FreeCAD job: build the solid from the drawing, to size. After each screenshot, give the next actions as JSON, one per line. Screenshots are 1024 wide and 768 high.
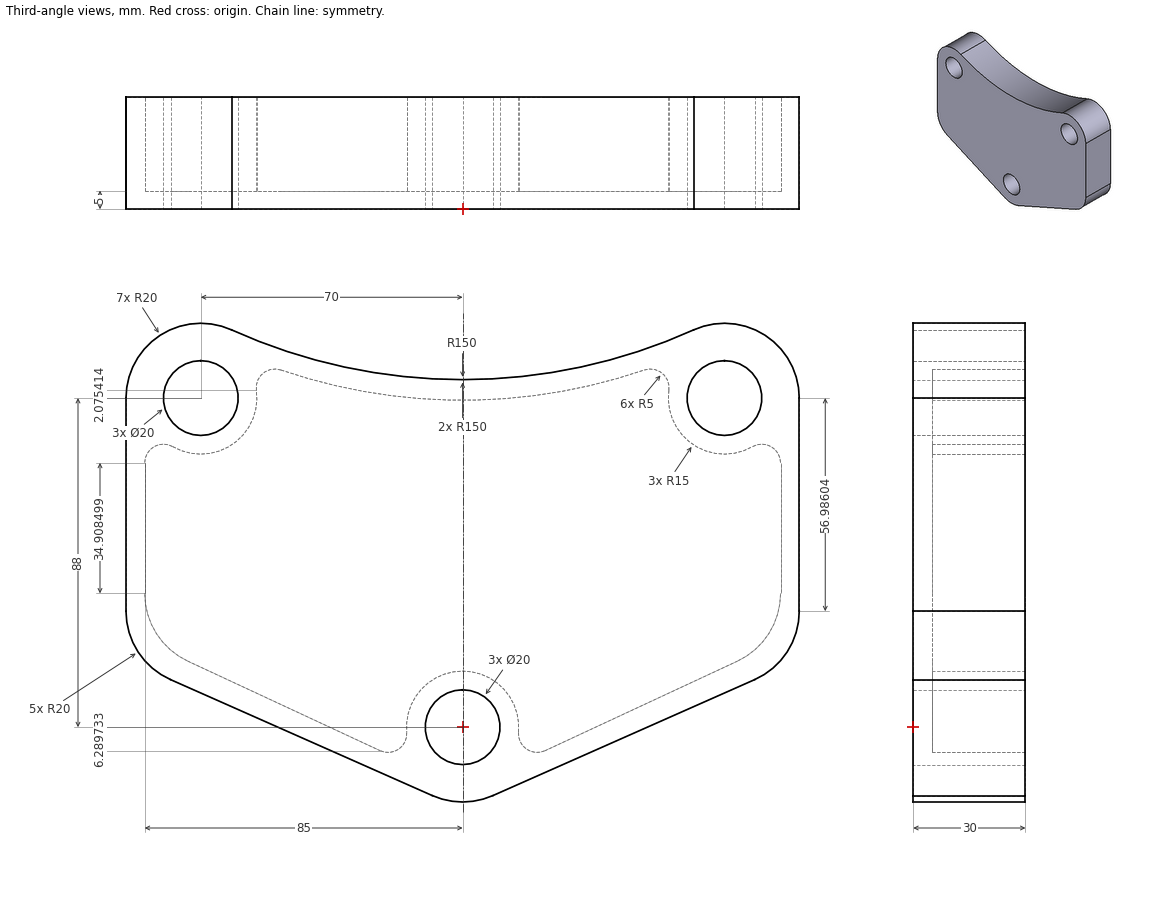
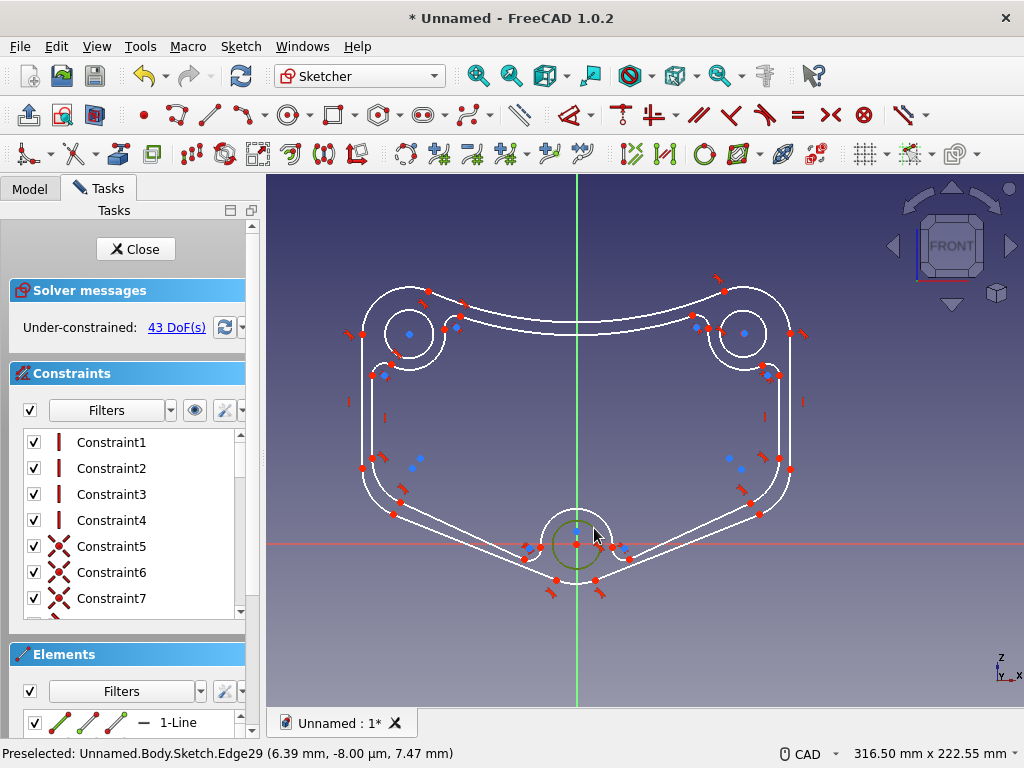
{"action": "left_click", "coordinate": [576, 584]}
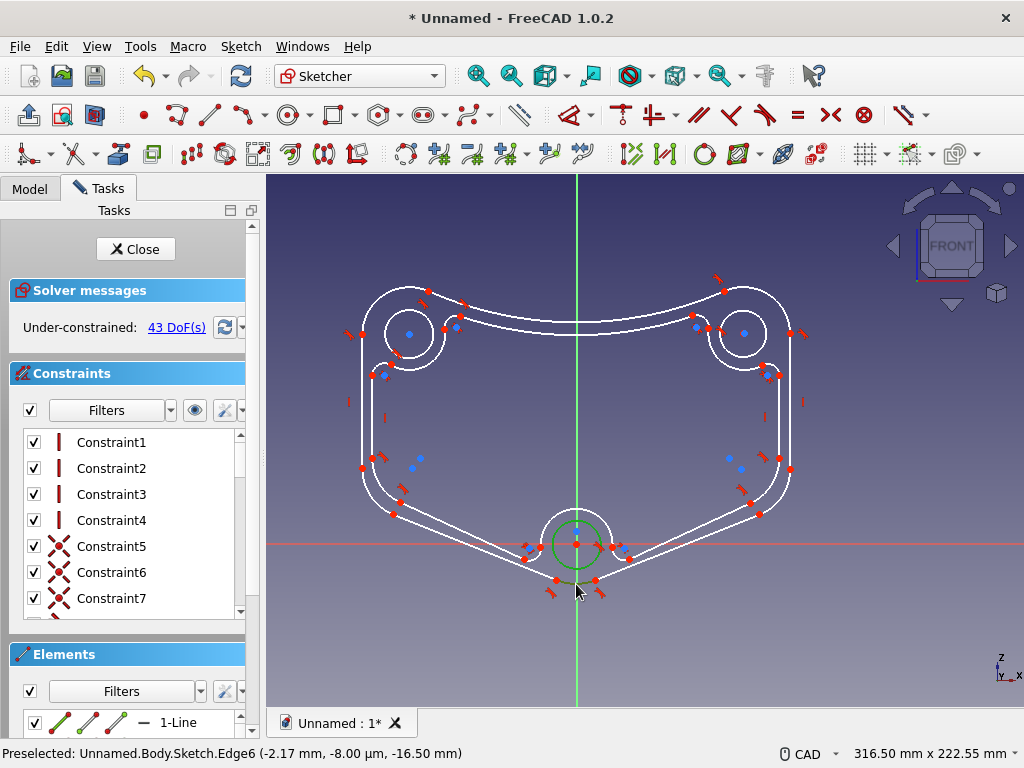
{"action": "left_click", "coordinate": [621, 116]}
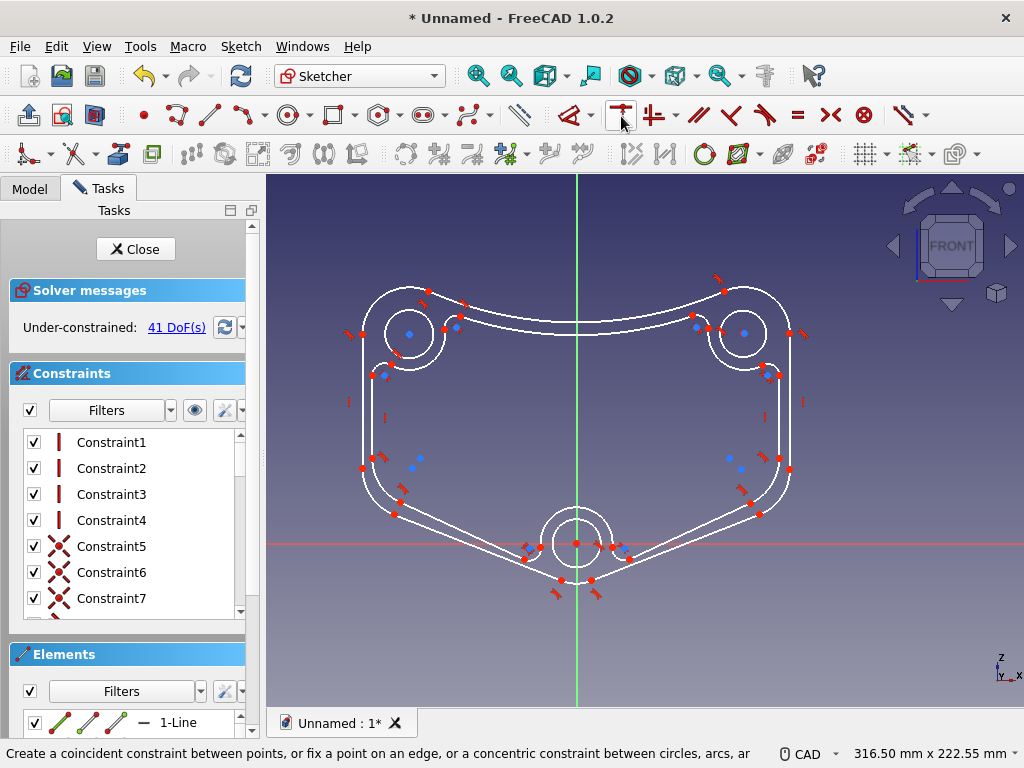
{"action": "left_click", "coordinate": [426, 317]}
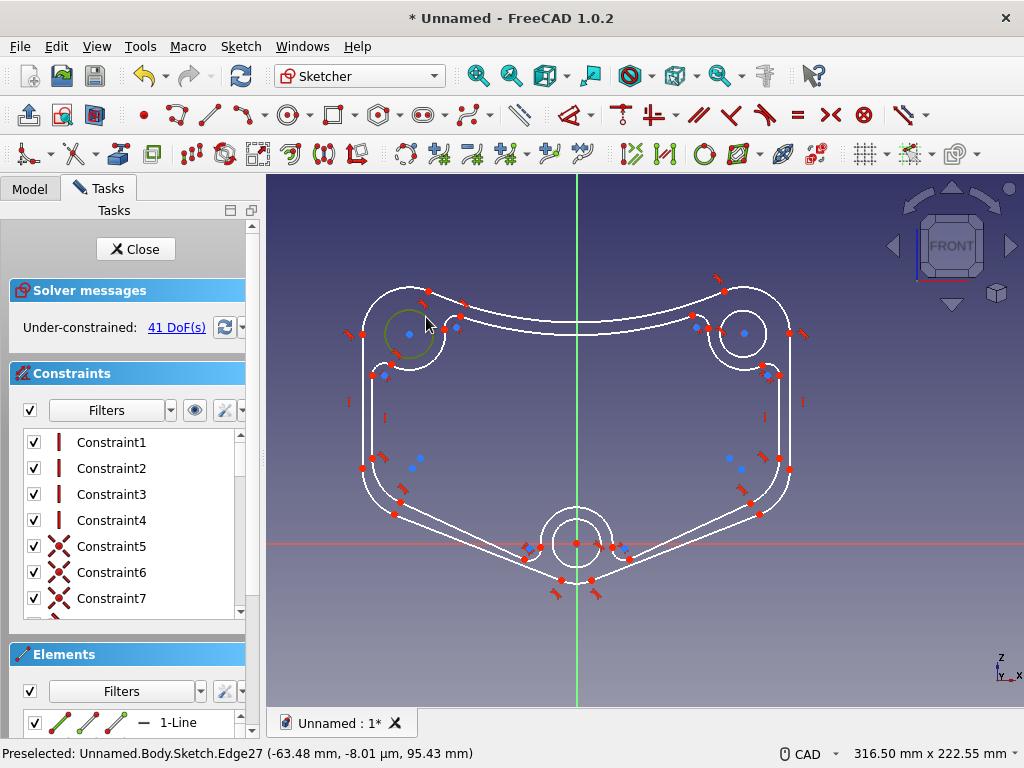
{"action": "left_click", "coordinate": [401, 288]}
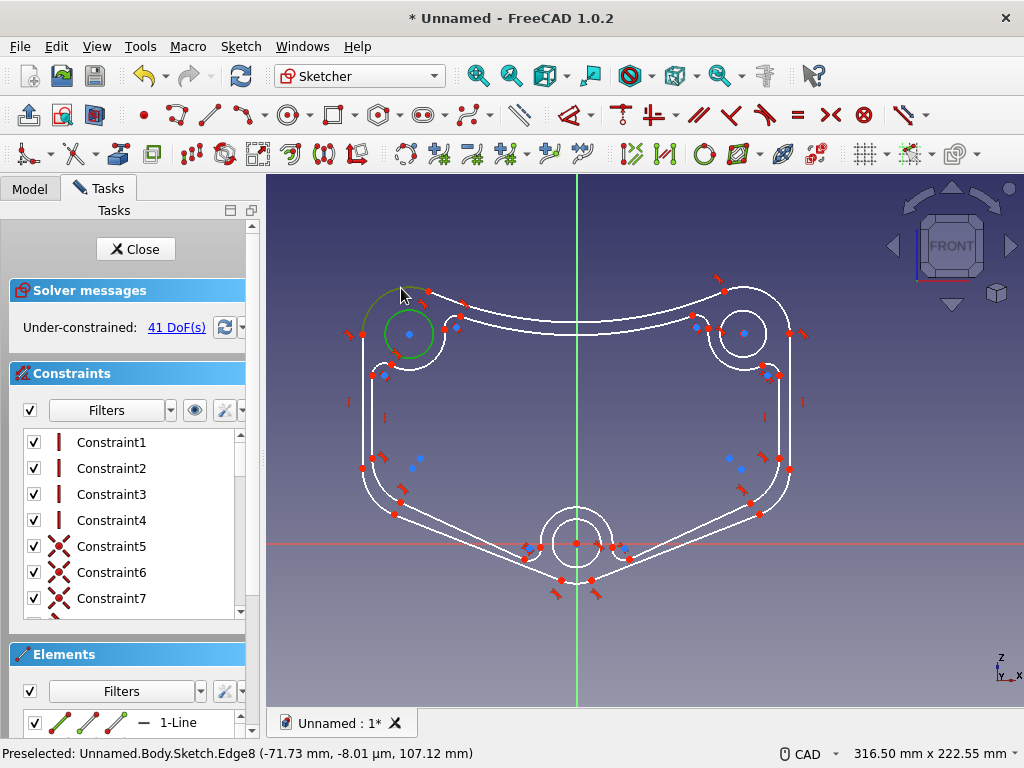
{"action": "left_click", "coordinate": [621, 116]}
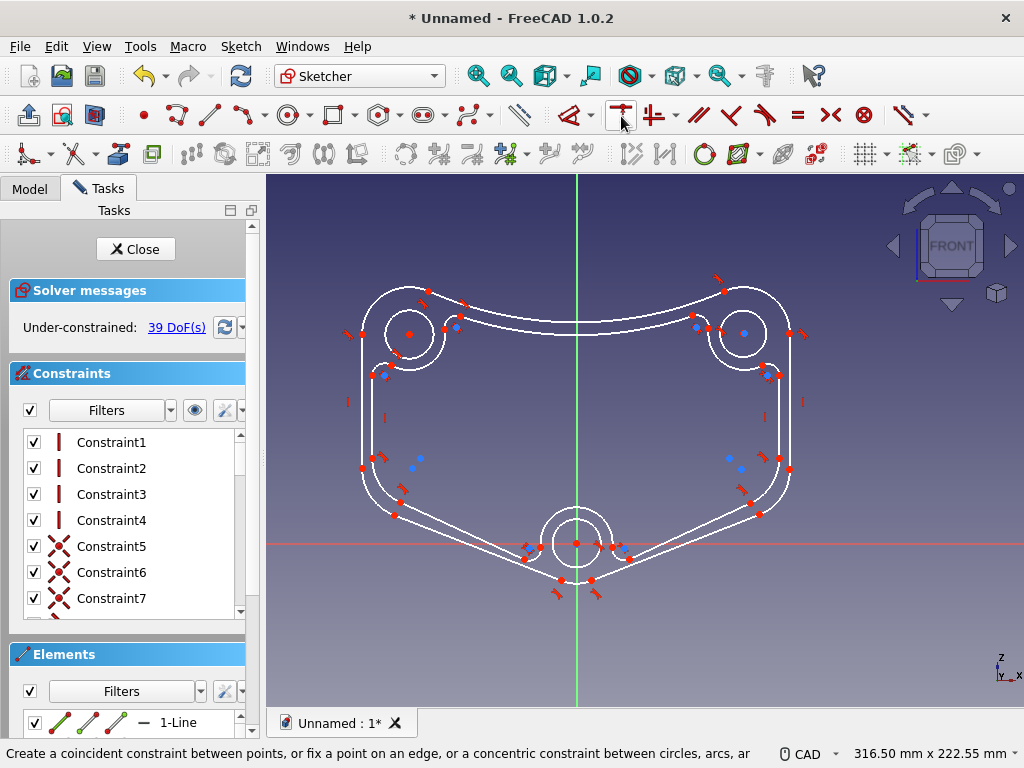
{"action": "left_click", "coordinate": [760, 317]}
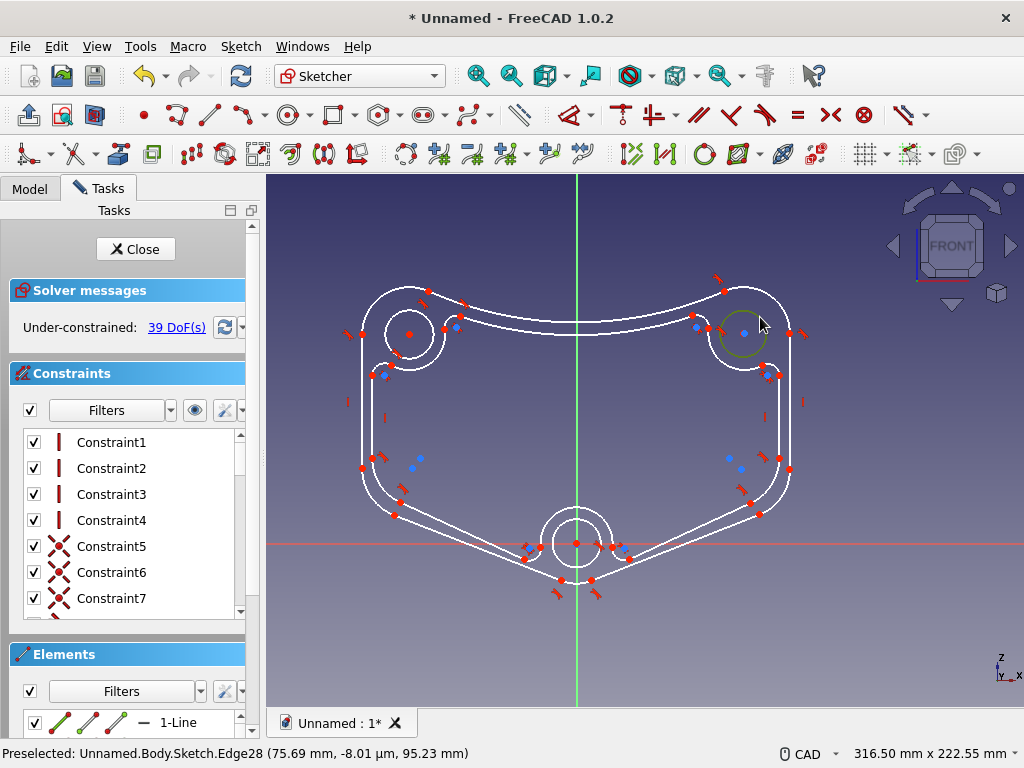
{"action": "left_click", "coordinate": [713, 352]}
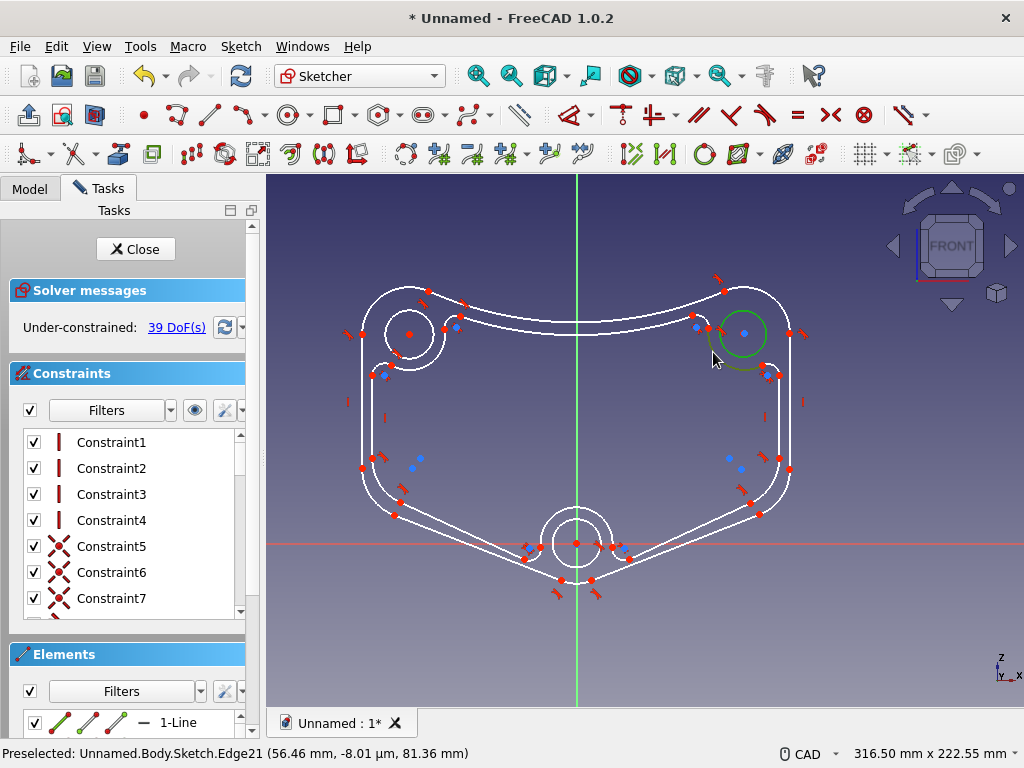
{"action": "left_click", "coordinate": [621, 116]}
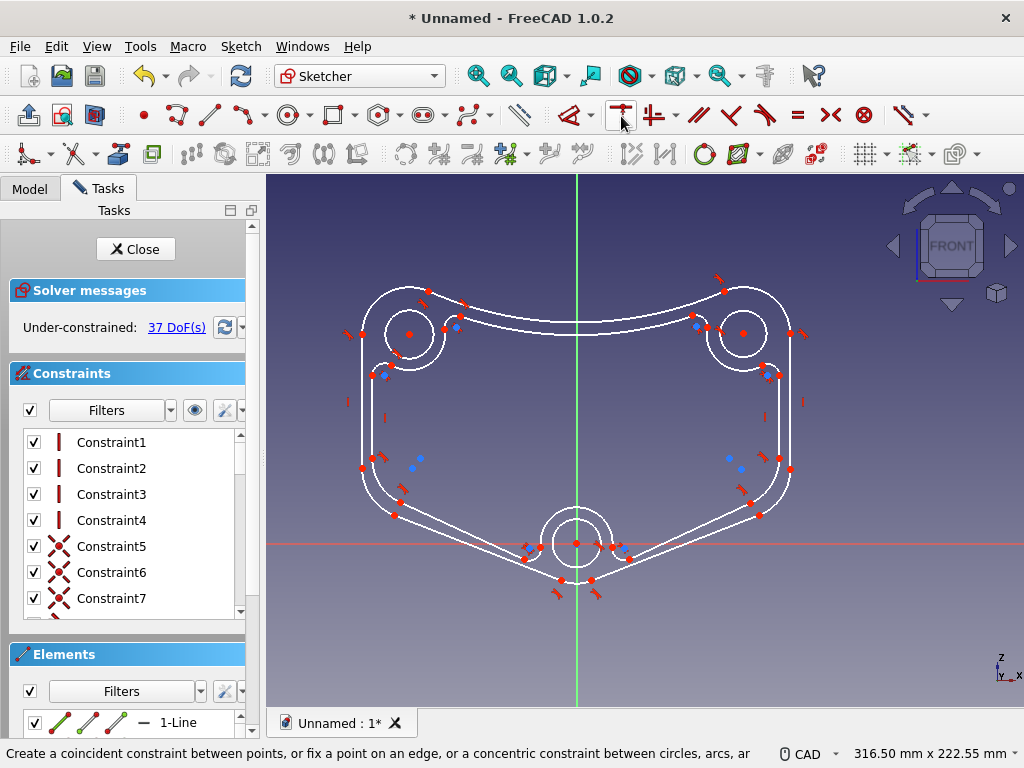
{"action": "scroll", "coordinate": [577, 544], "scroll_direction": "up", "scroll_amount": 7}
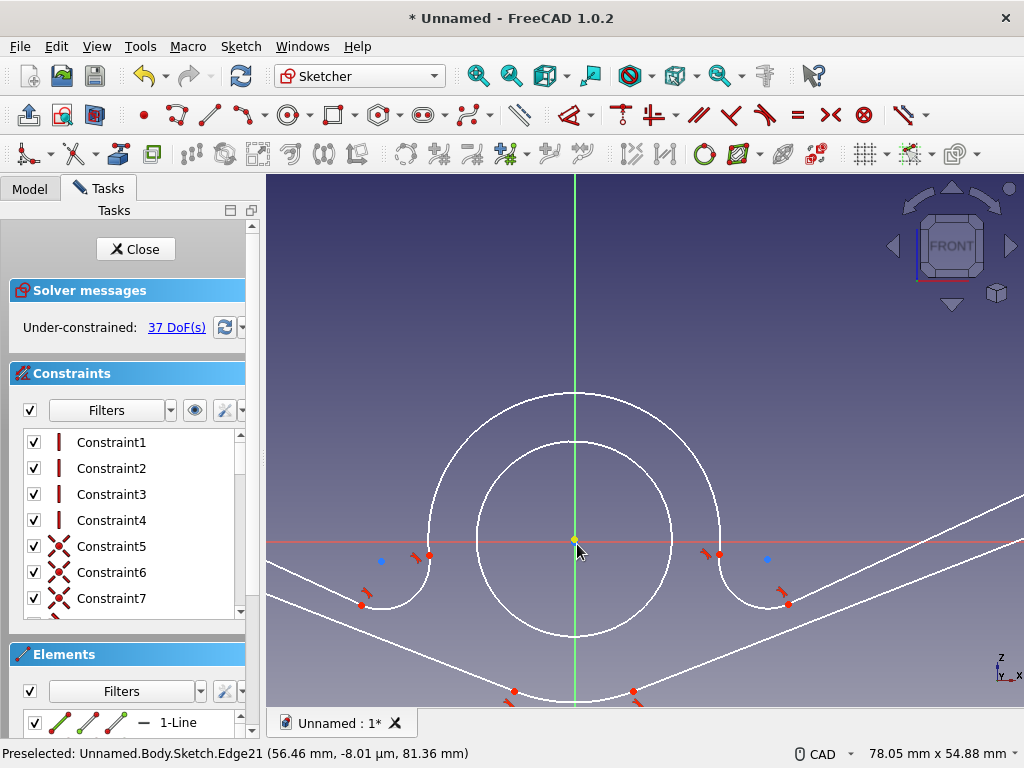
{"action": "left_click_drag", "start_coordinate": [564, 529], "coordinate": [585, 552]}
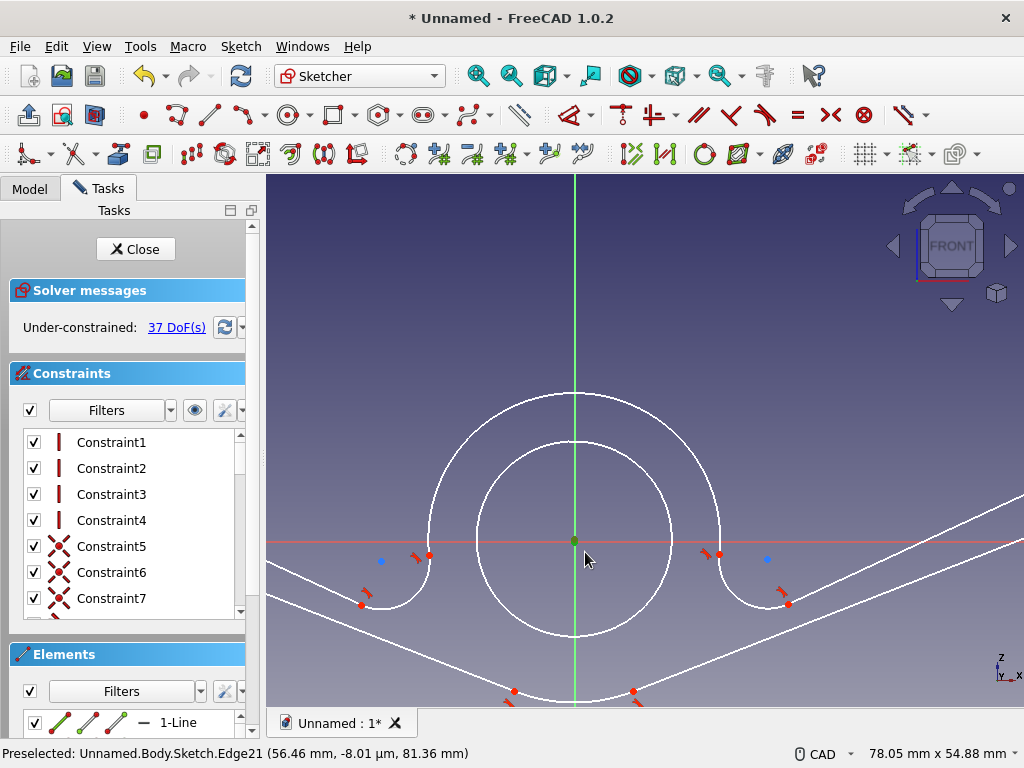
{"action": "left_click", "coordinate": [621, 116]}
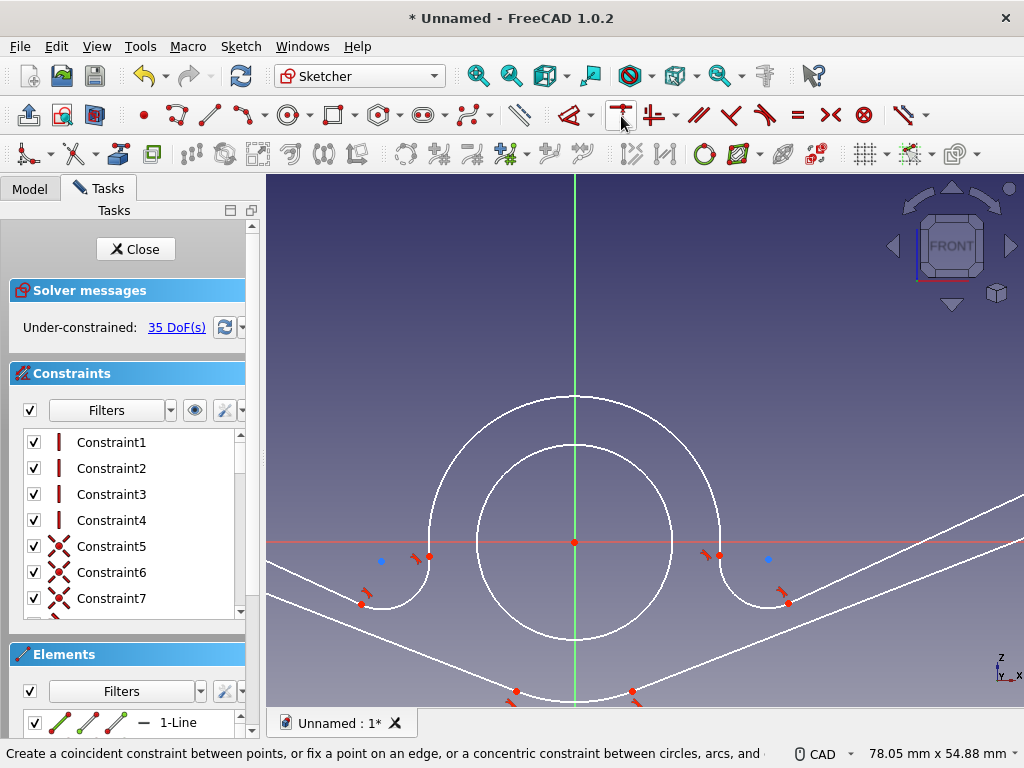
{"action": "scroll", "coordinate": [577, 544], "scroll_direction": "down", "scroll_amount": 7}